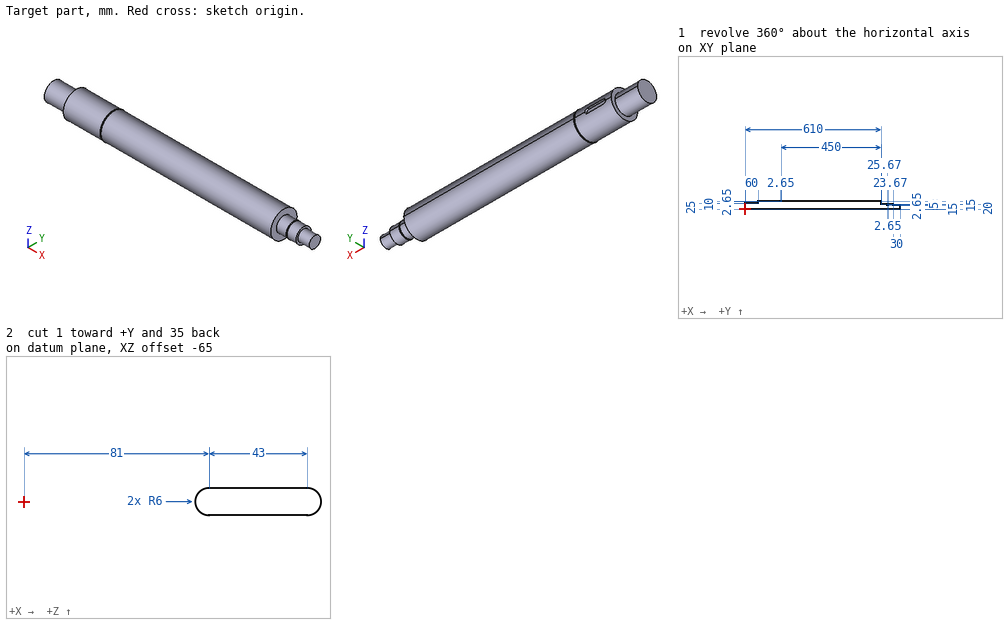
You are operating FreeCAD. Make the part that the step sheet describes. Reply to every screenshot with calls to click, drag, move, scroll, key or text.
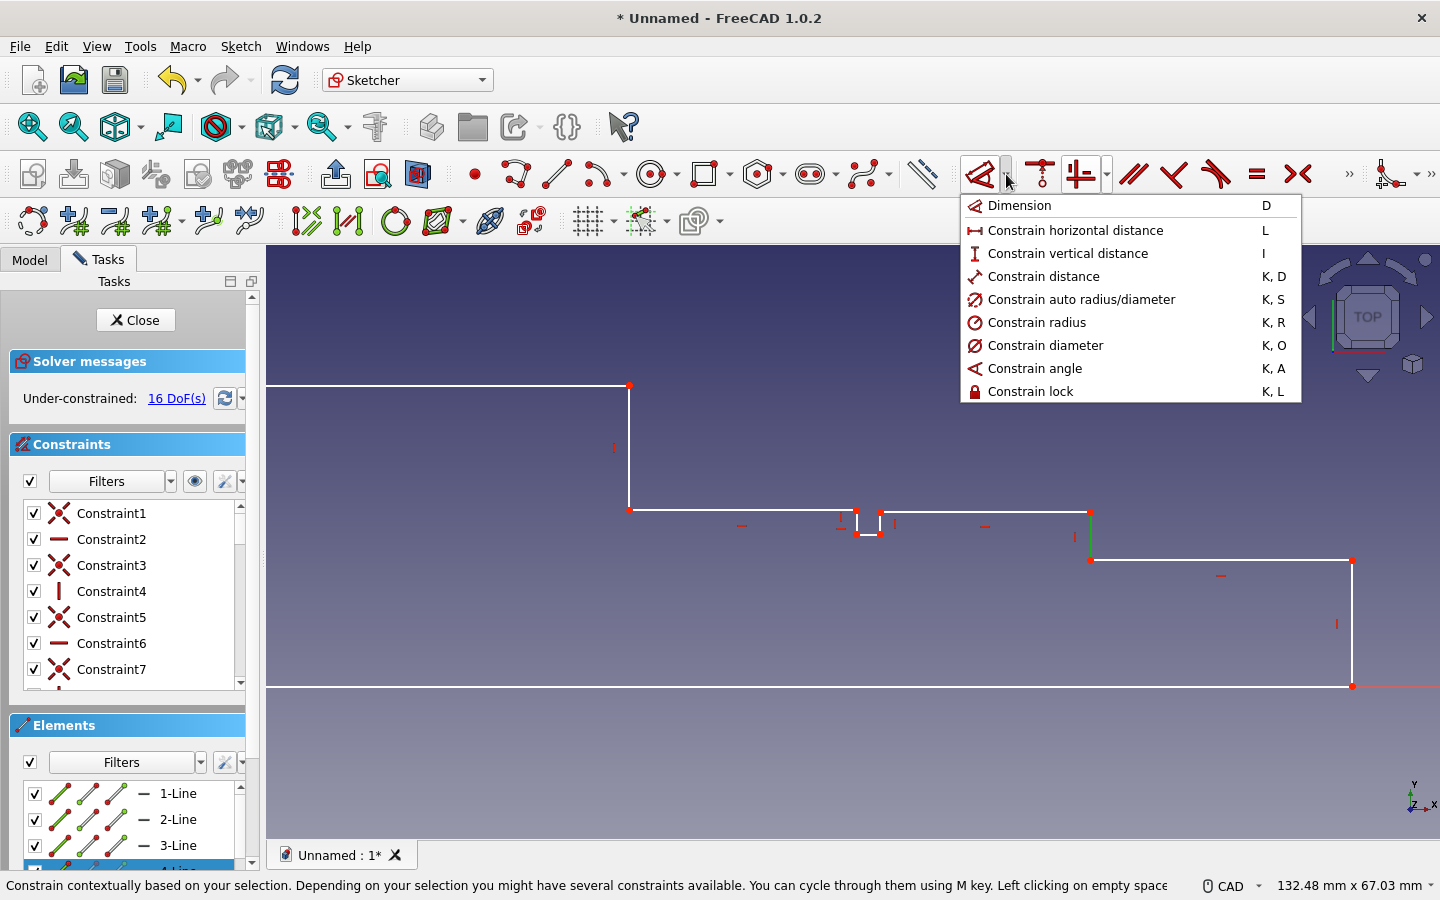
click(1131, 254)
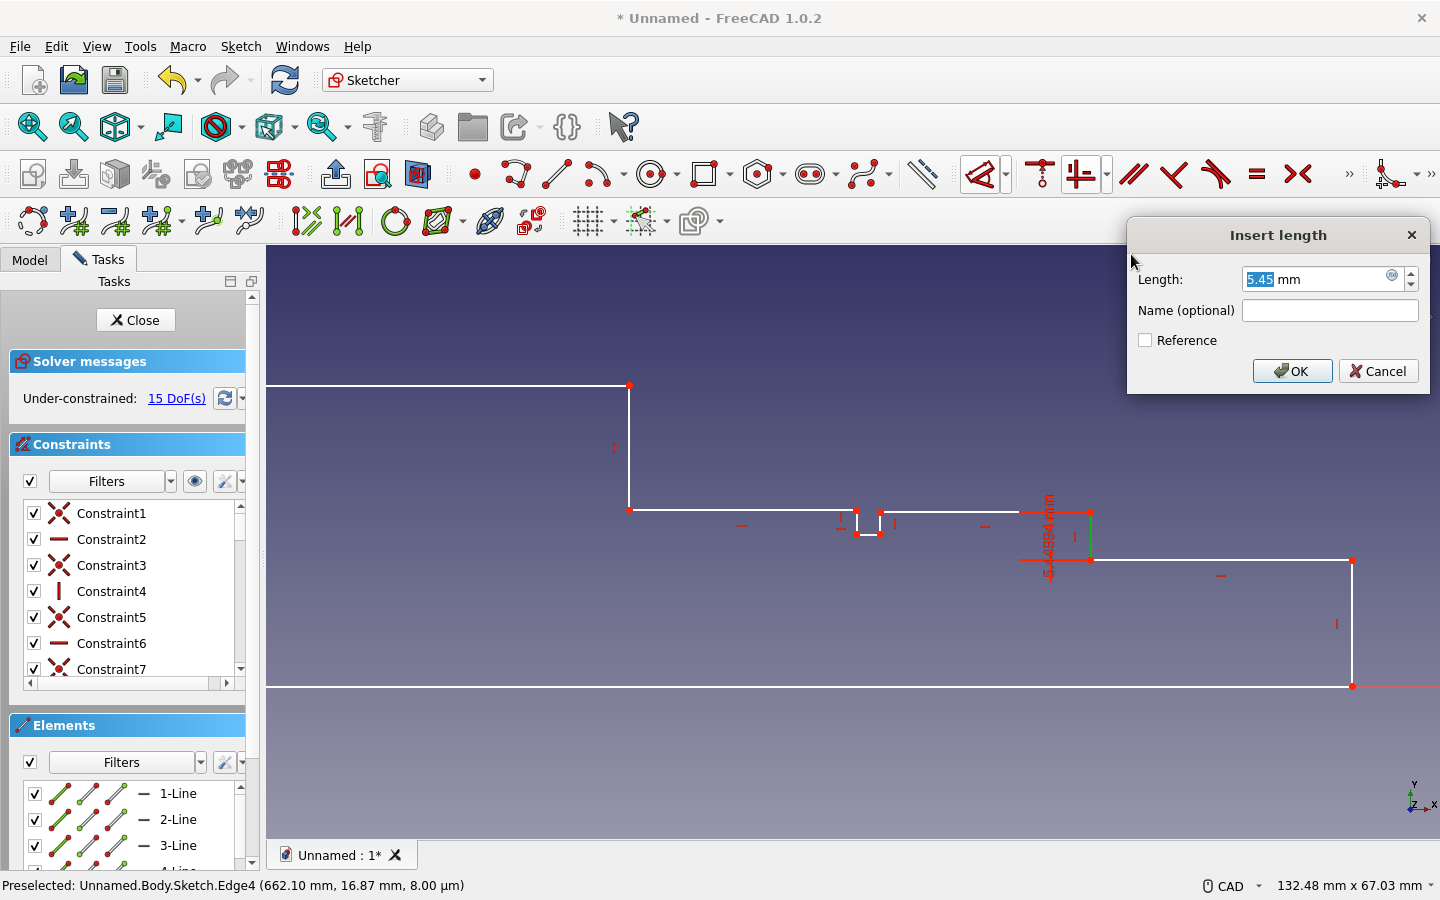
text(5)
key(Return)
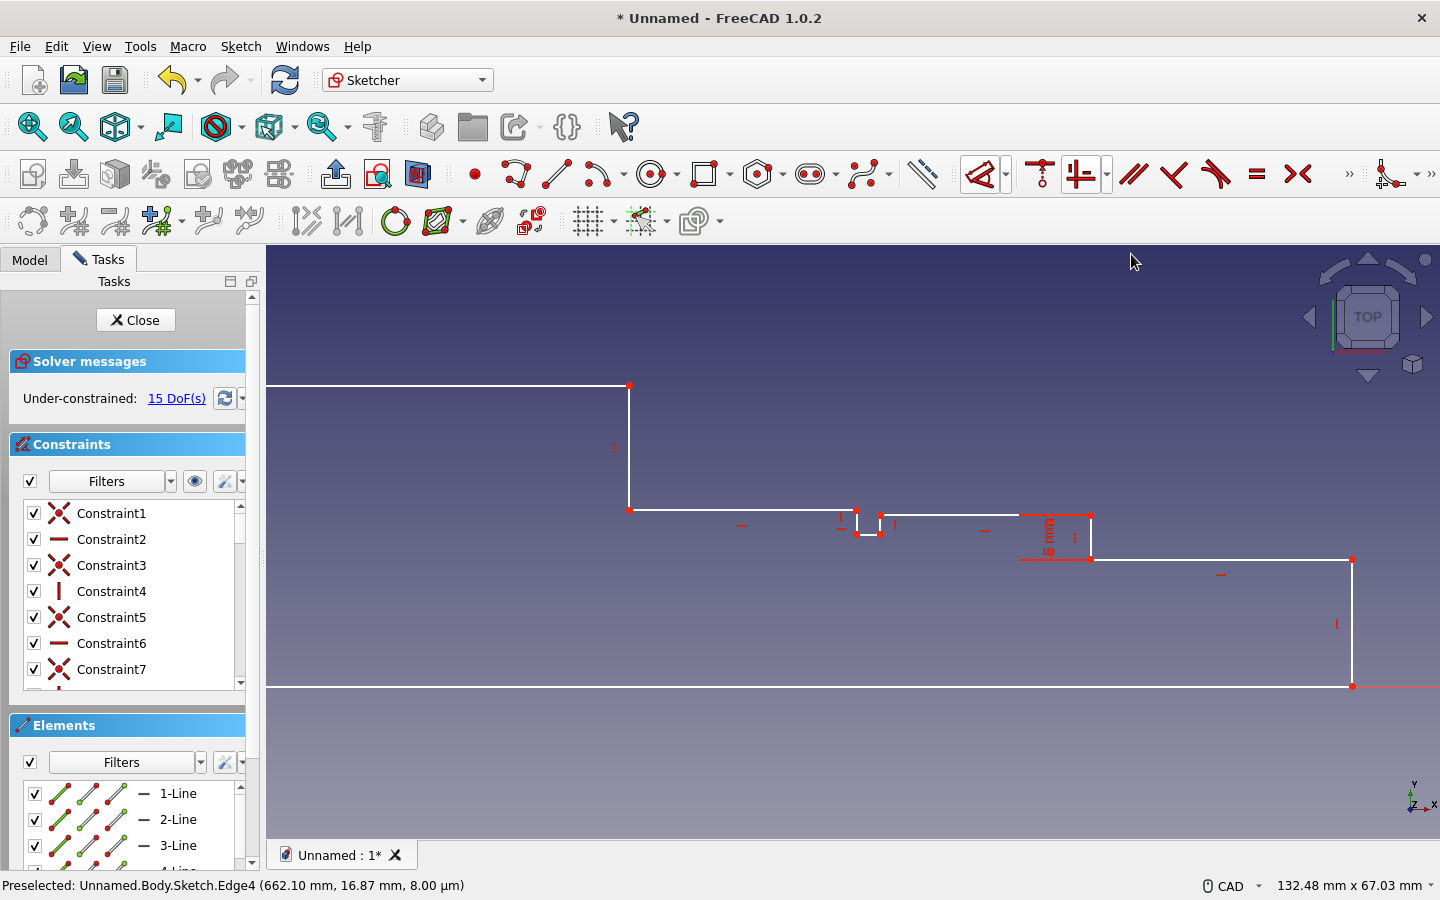
scroll(1095, 543, down, 11)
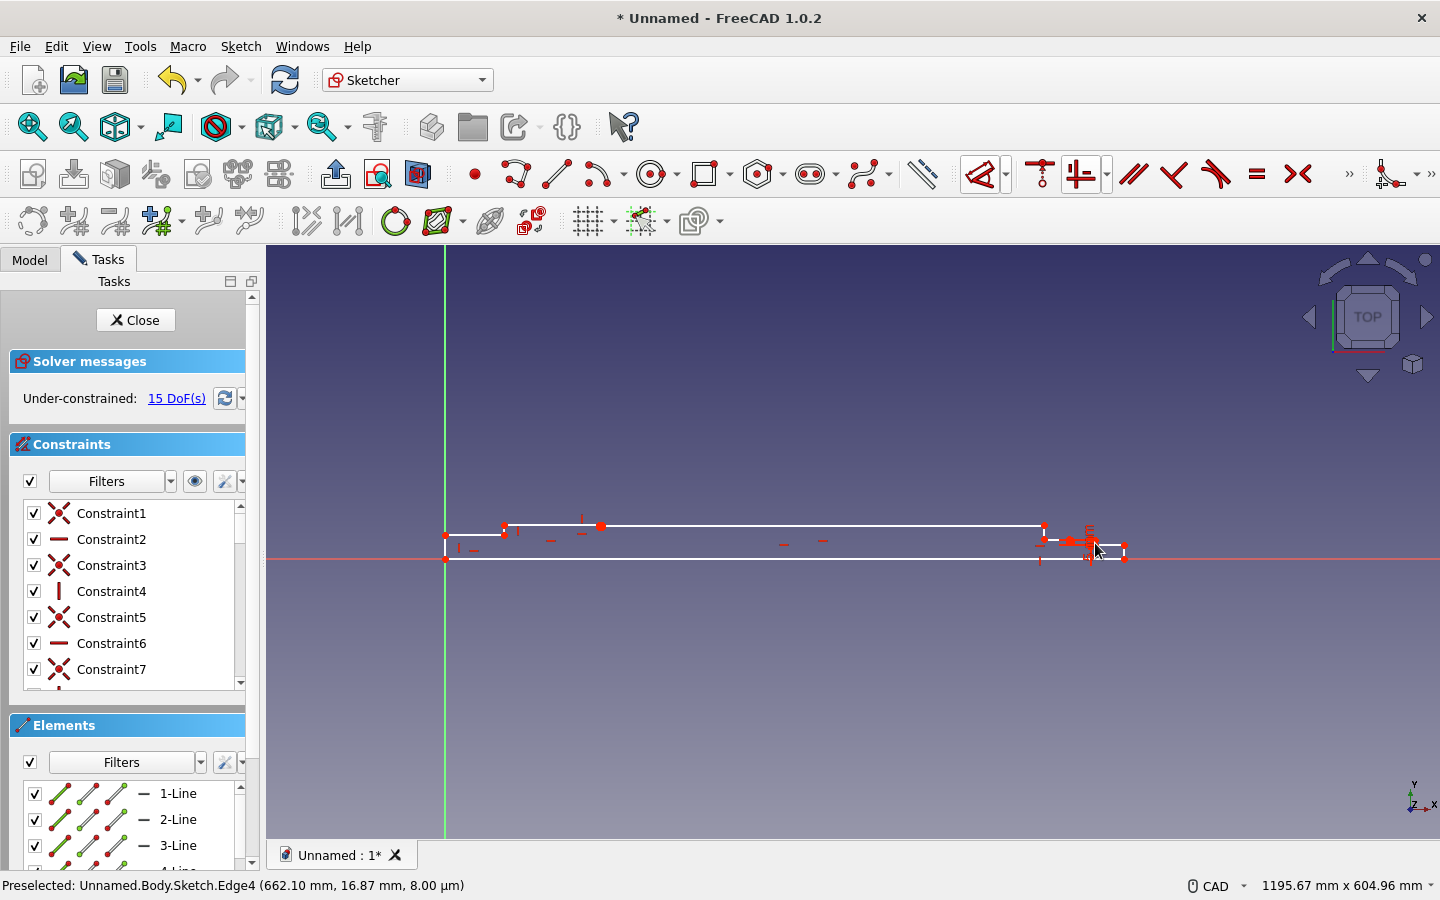
scroll(1124, 555, up, 6)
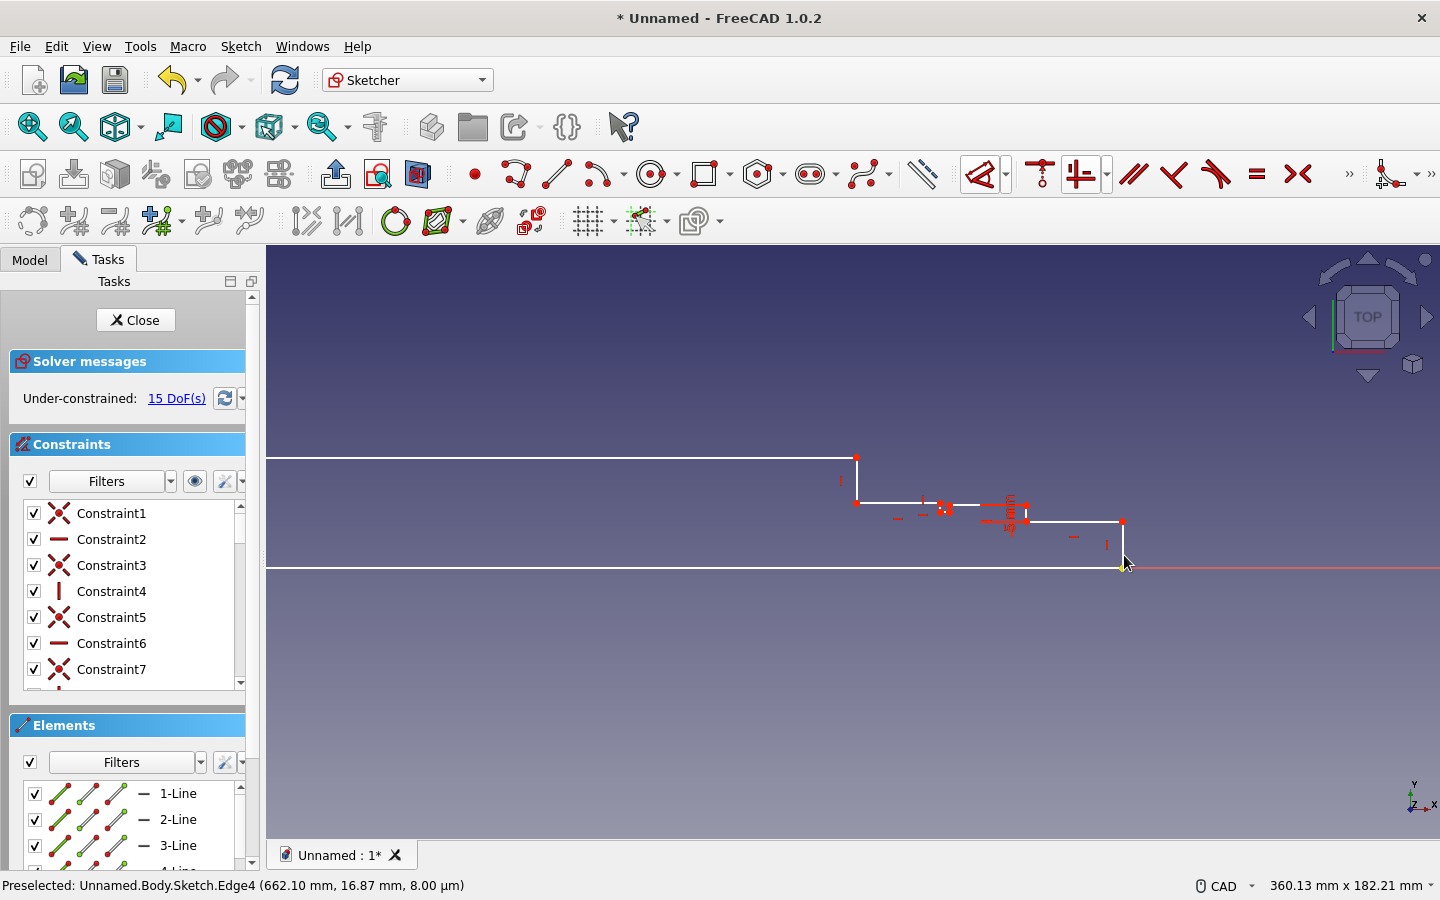
click(1123, 554)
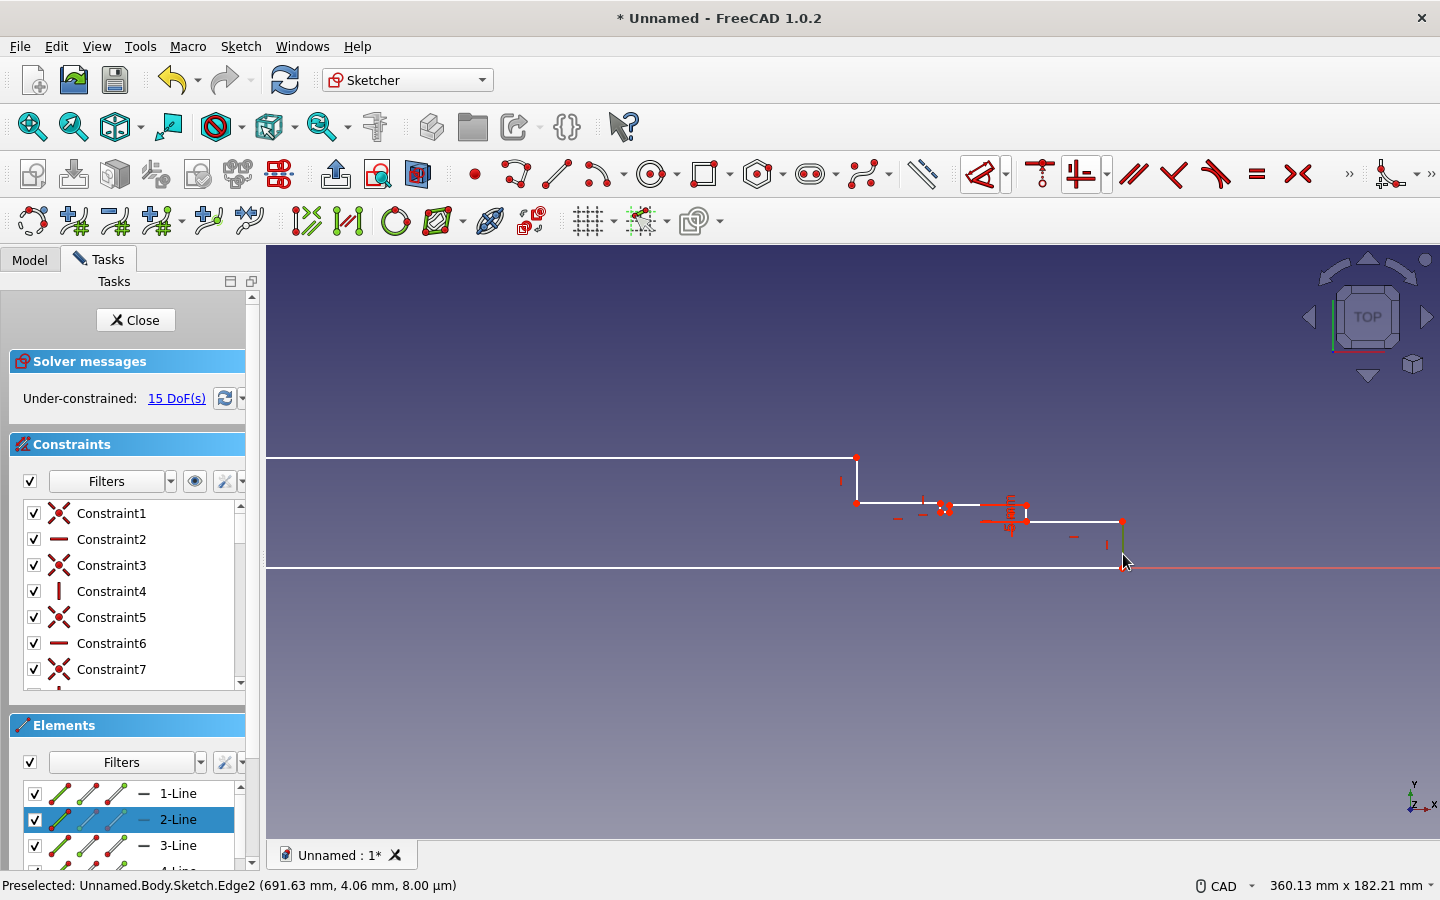
key(i)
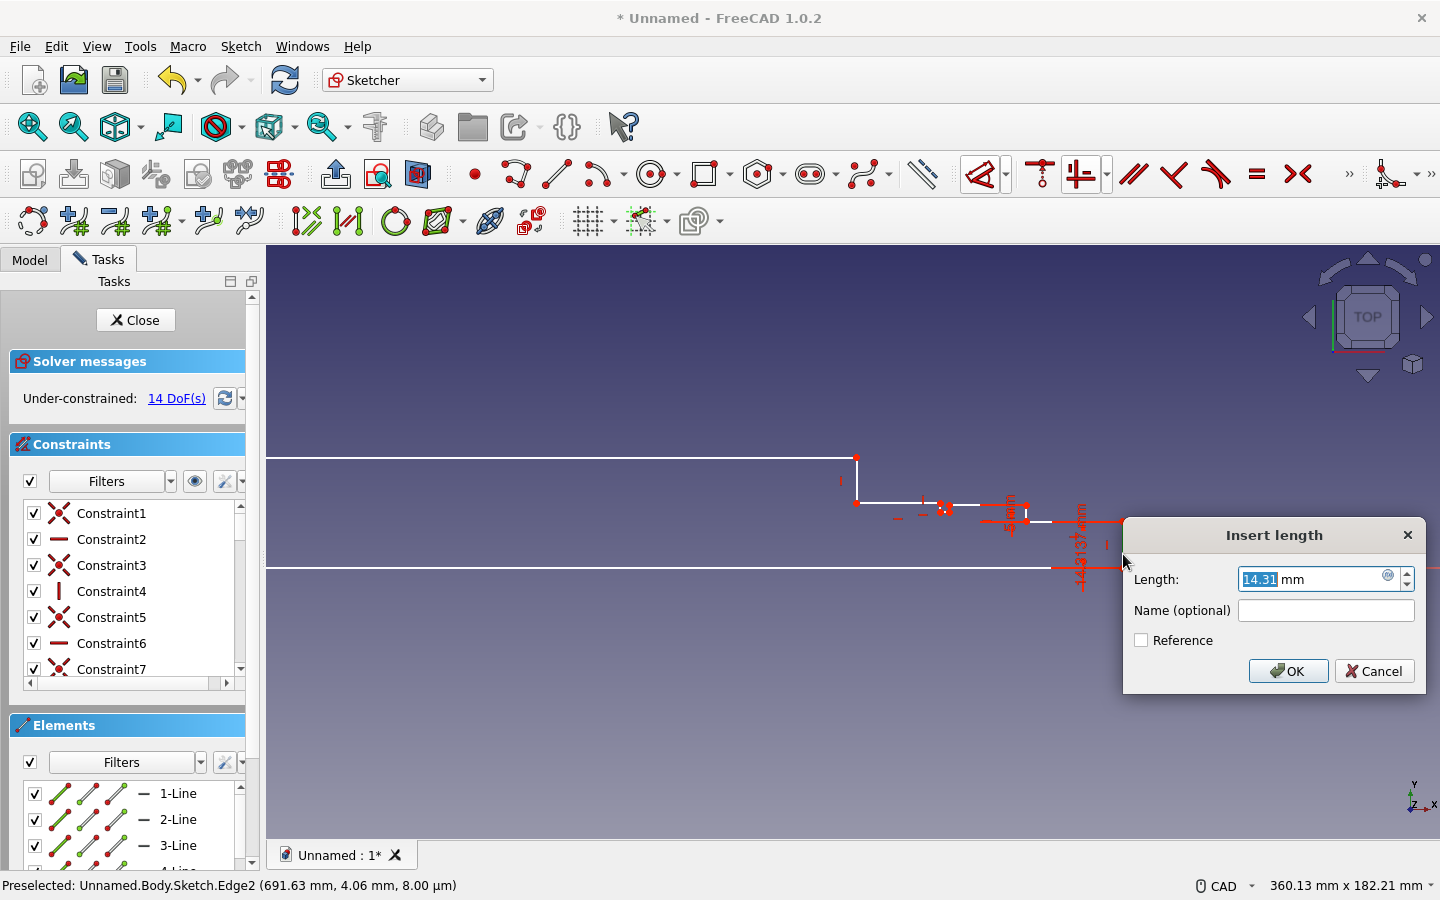
text(15)
key(Return)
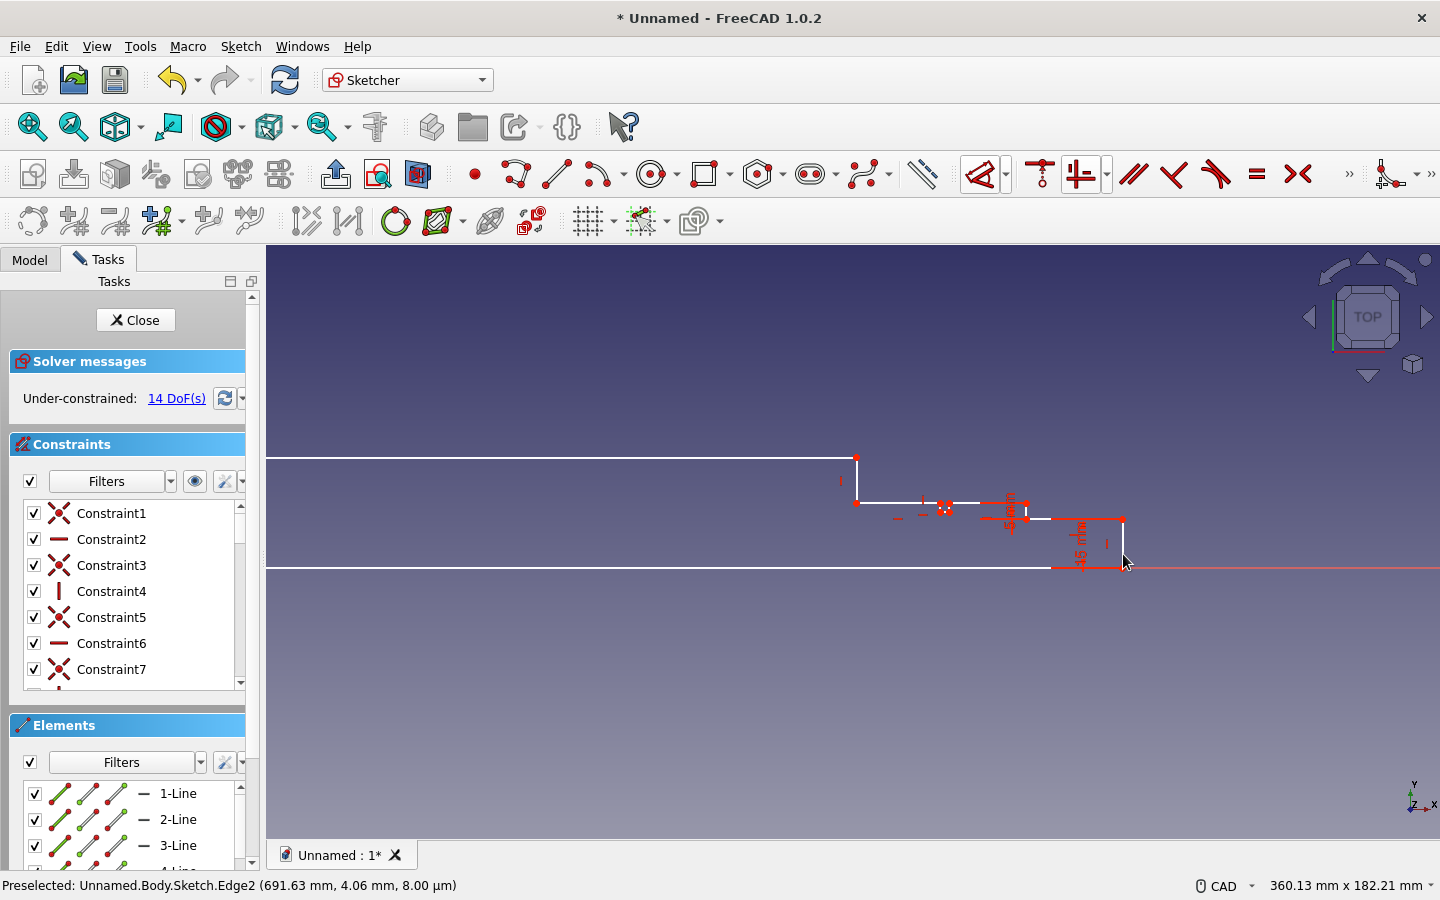
click(1094, 519)